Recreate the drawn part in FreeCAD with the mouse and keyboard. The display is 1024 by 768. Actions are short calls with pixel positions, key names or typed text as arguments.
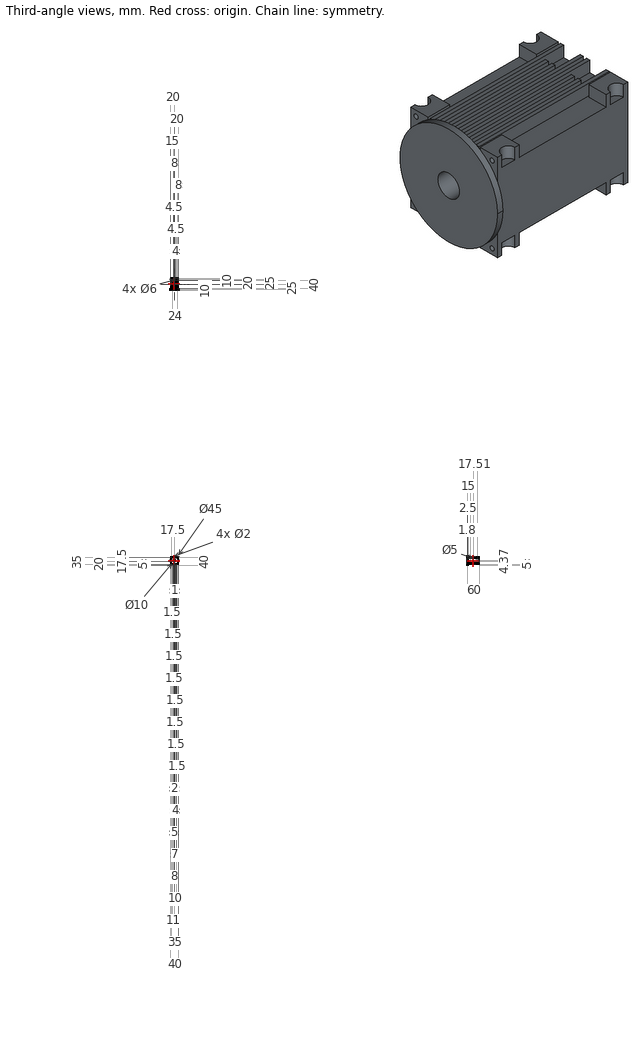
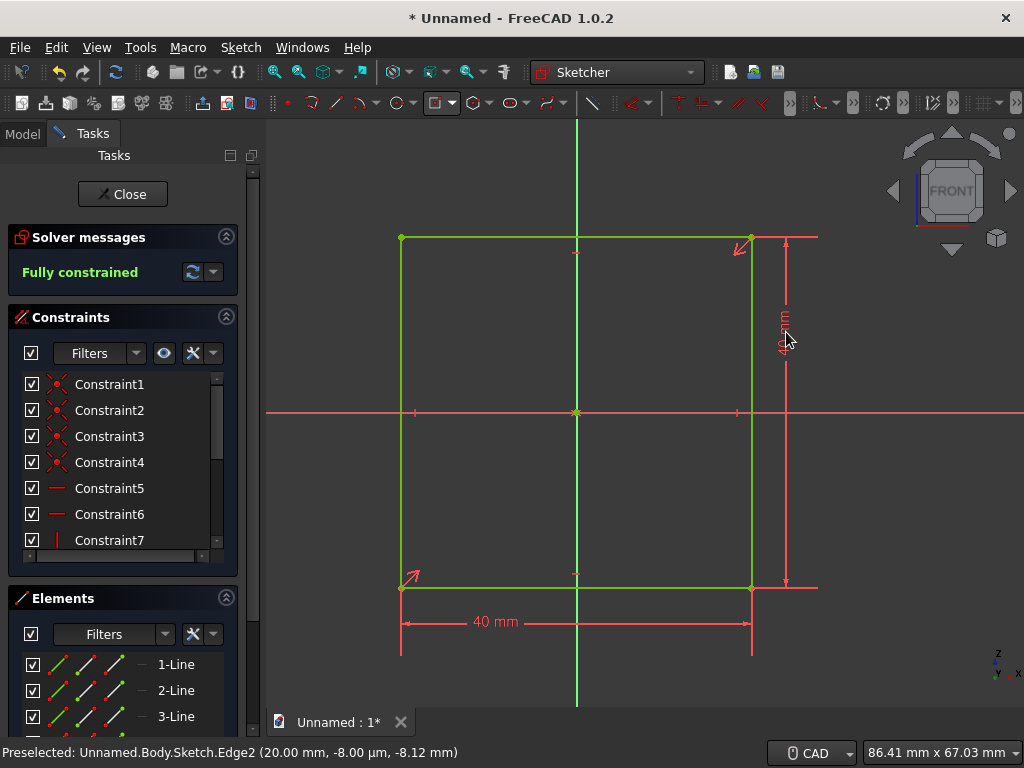
click(123, 194)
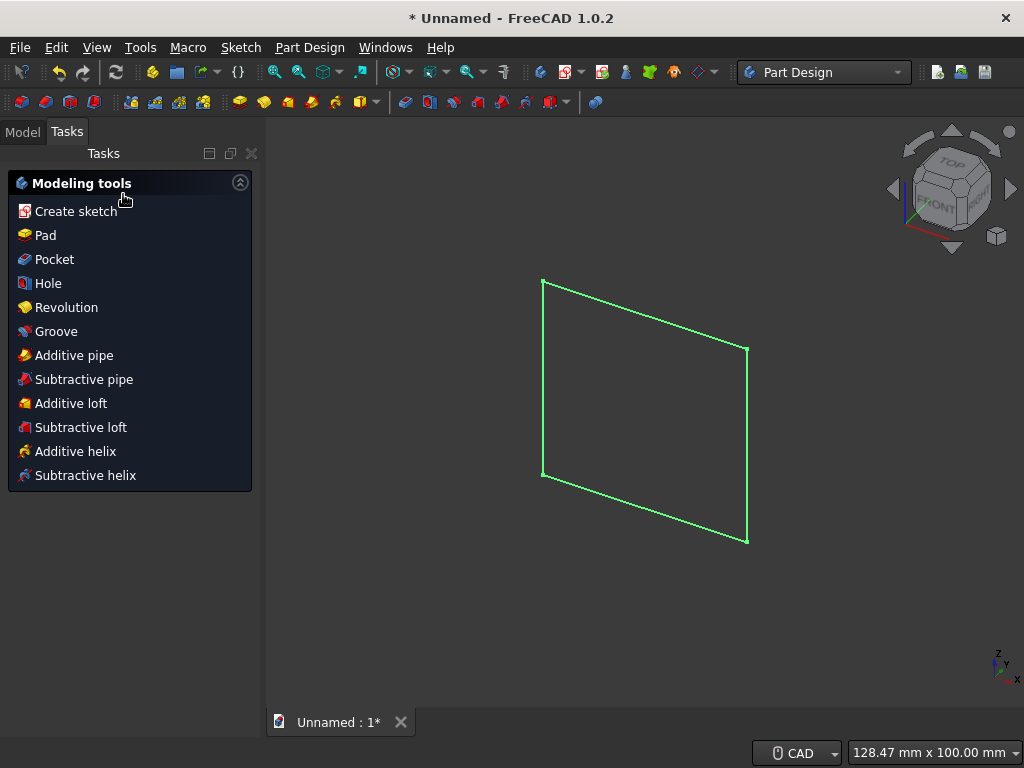
click(240, 102)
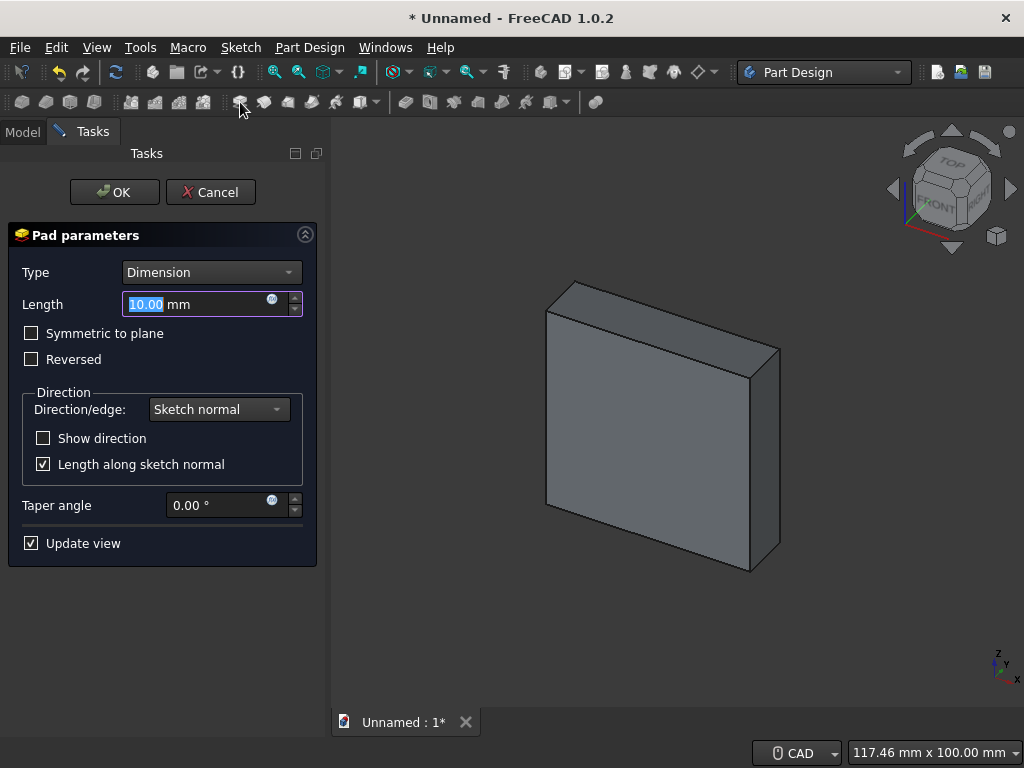
text(60)
key(Tab)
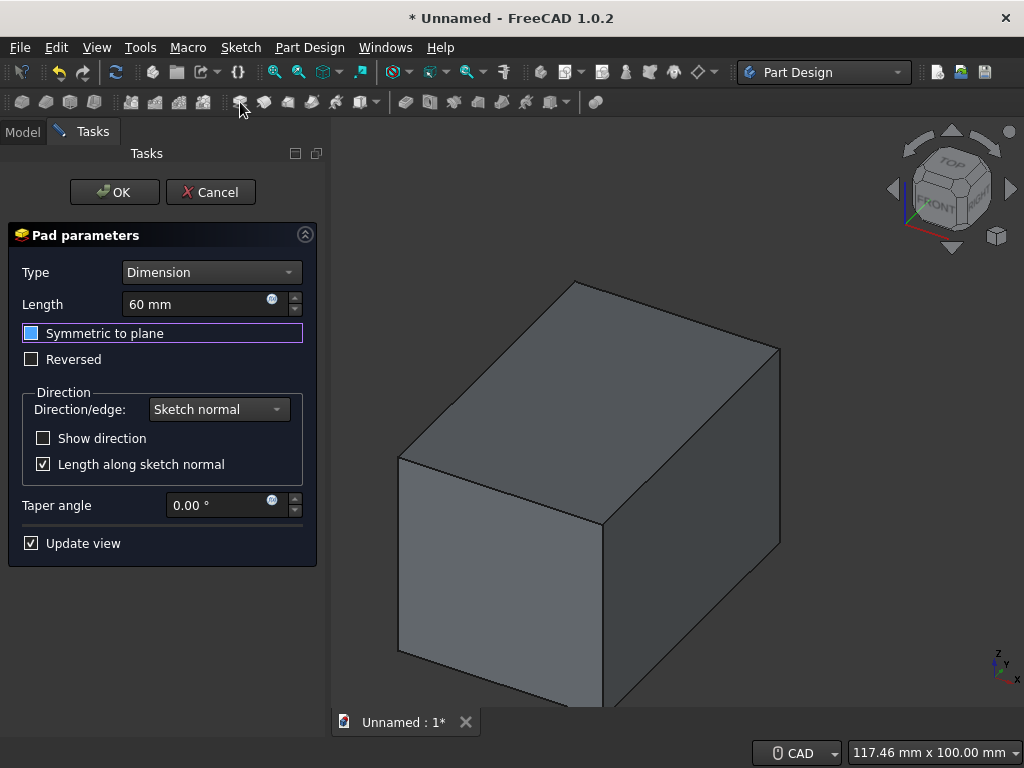
click(30, 333)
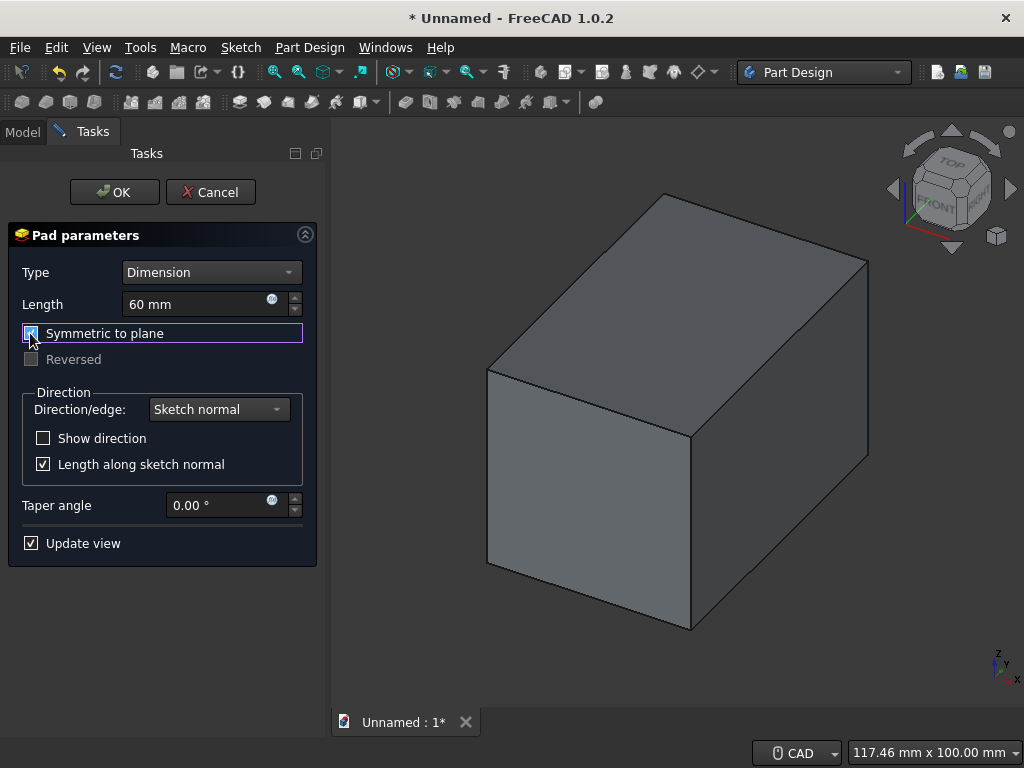
click(115, 192)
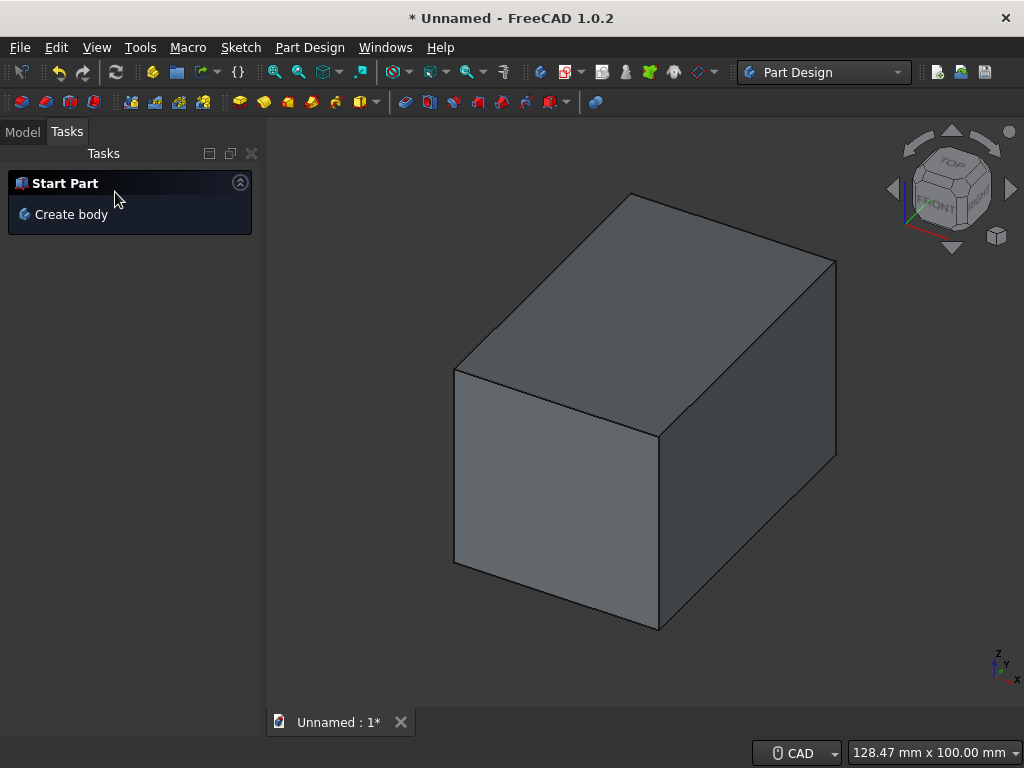
key(5)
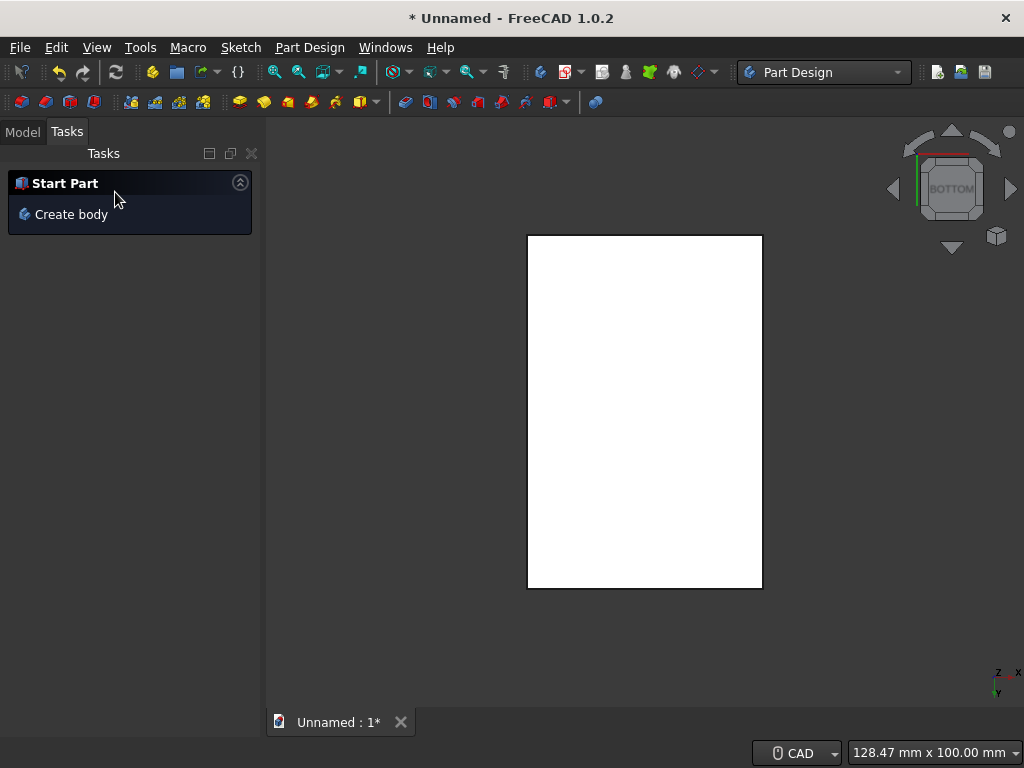
click(645, 462)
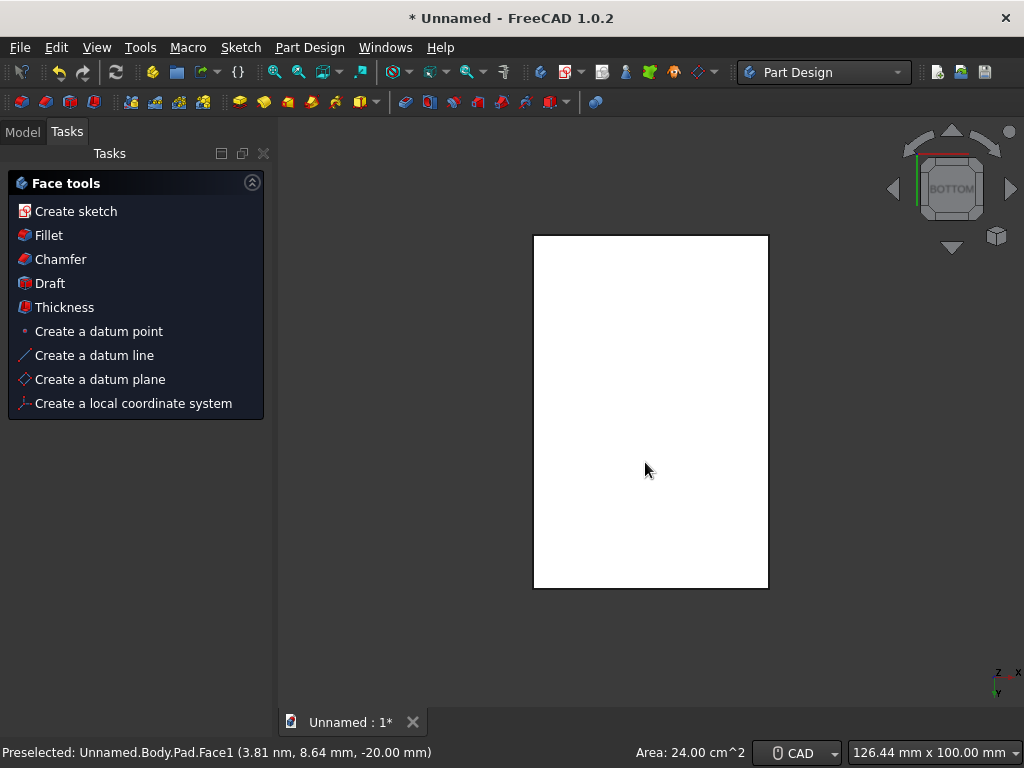
click(566, 72)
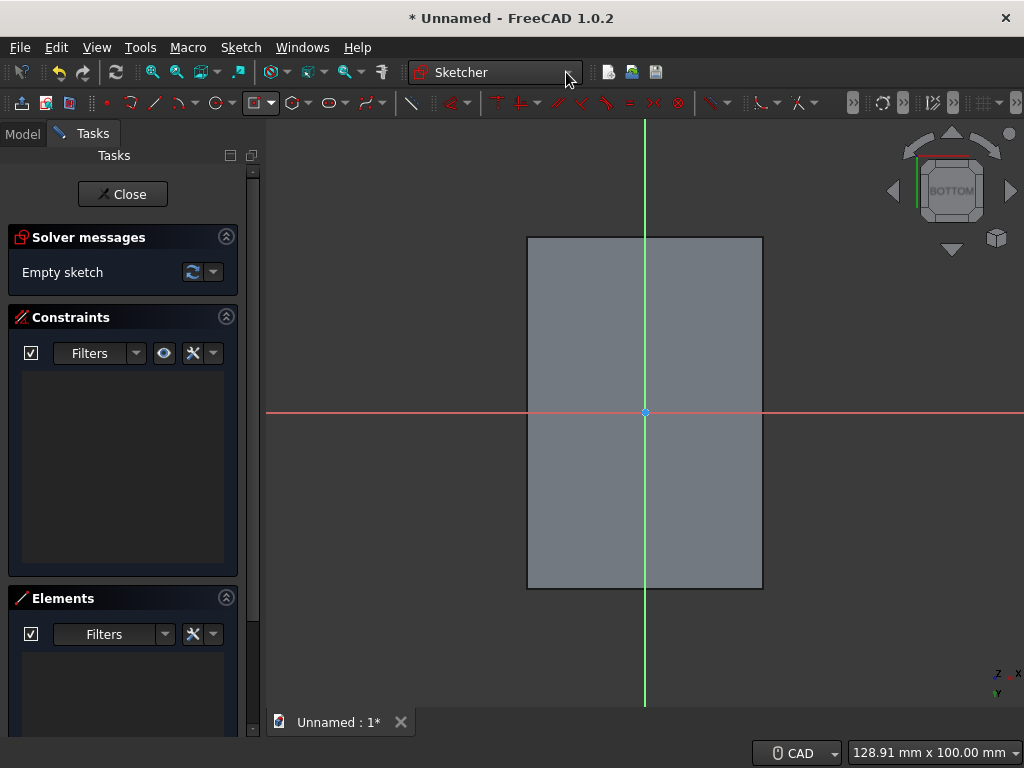
click(132, 104)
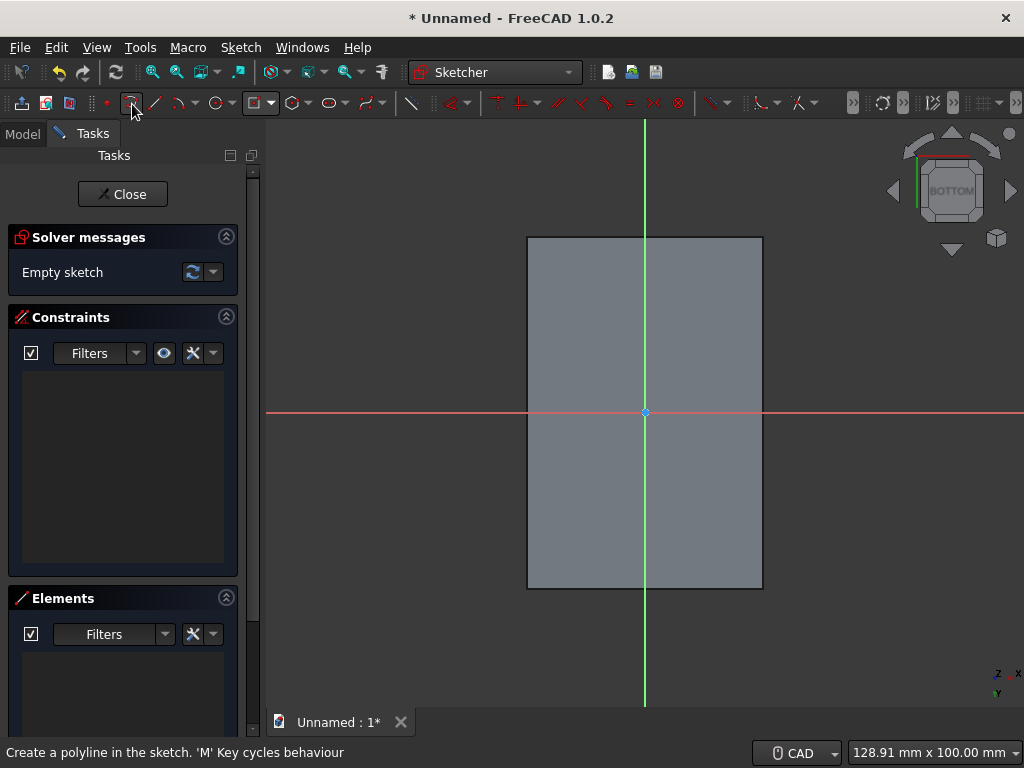
click(716, 531)
click(763, 531)
click(763, 295)
click(716, 295)
click(716, 237)
click(574, 237)
click(574, 295)
click(527, 295)
click(527, 531)
click(574, 531)
click(574, 589)
click(716, 589)
click(716, 532)
key(Escape)
key(Escape)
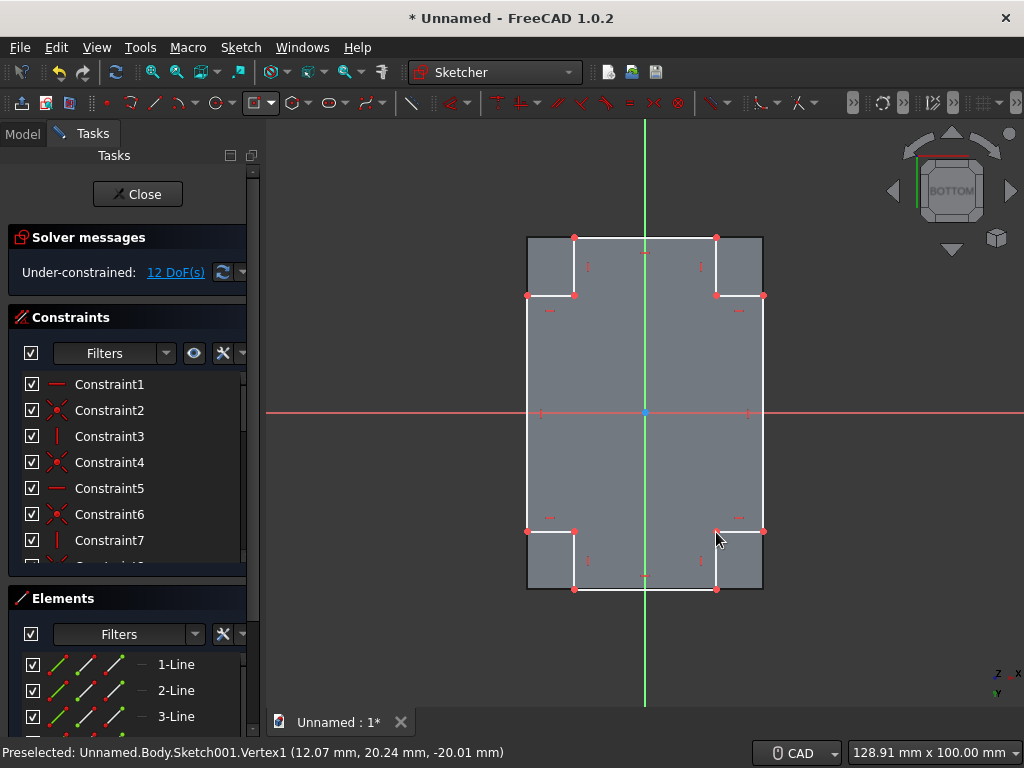
click(716, 532)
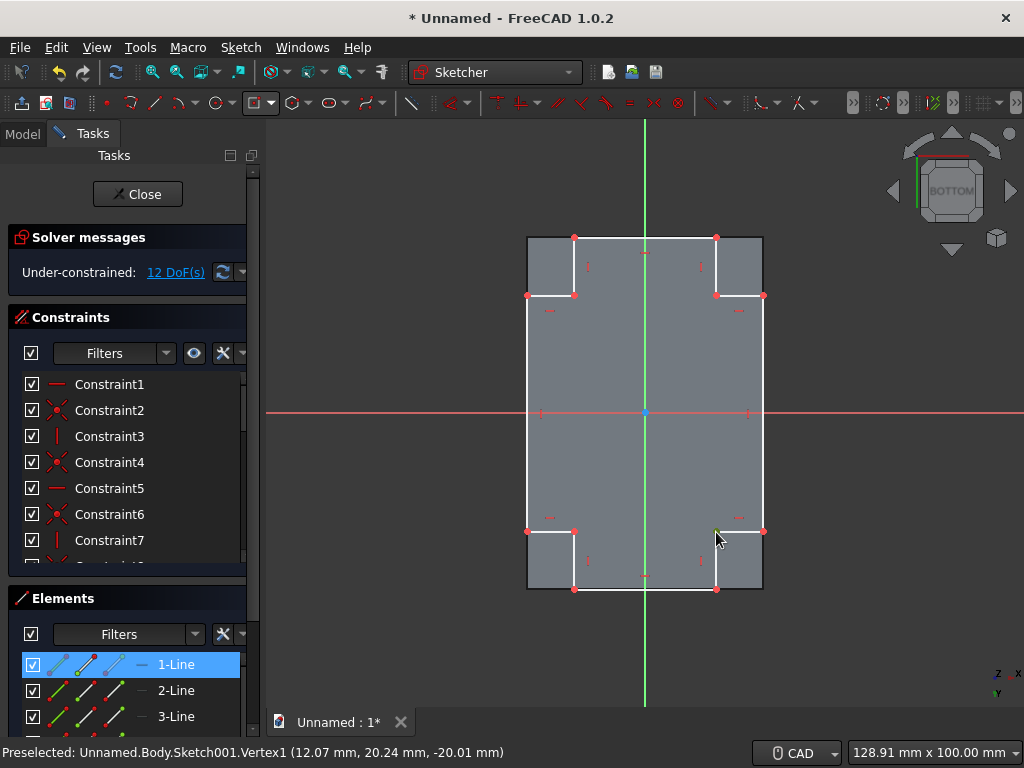
click(716, 296)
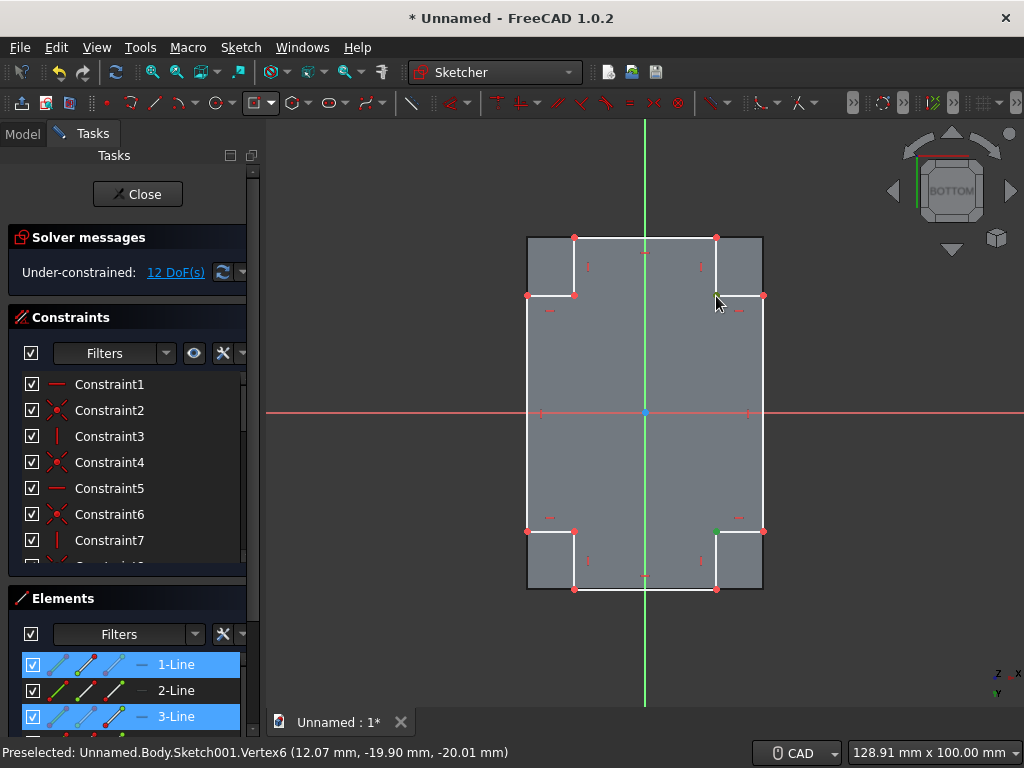
click(334, 413)